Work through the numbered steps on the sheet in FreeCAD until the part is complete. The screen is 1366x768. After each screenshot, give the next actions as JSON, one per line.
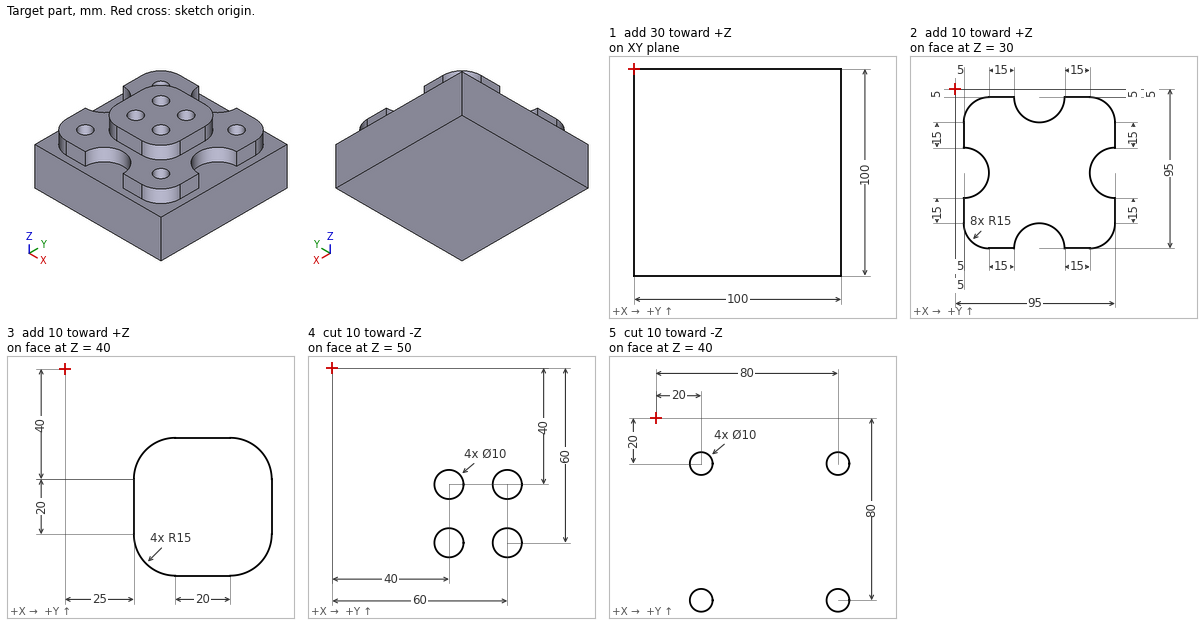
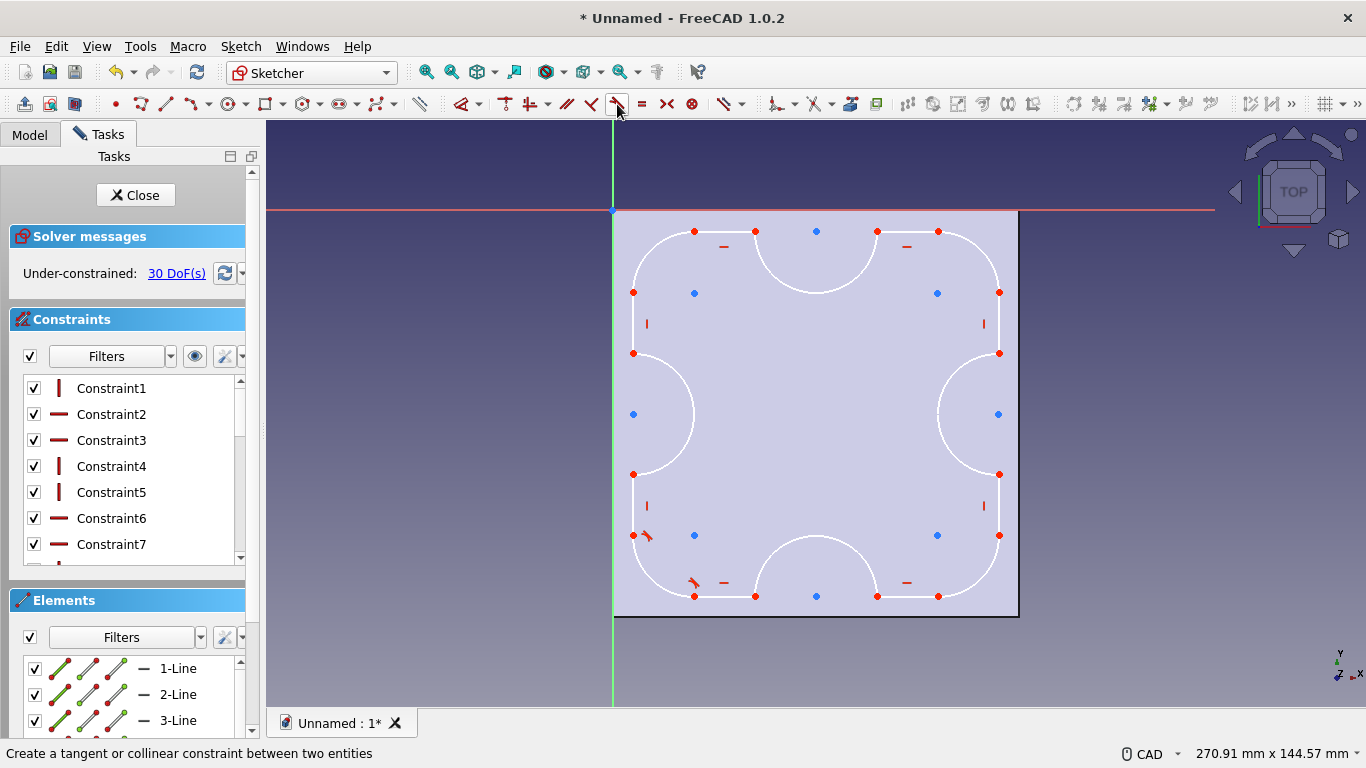
{"action": "left_click", "coordinate": [895, 597]}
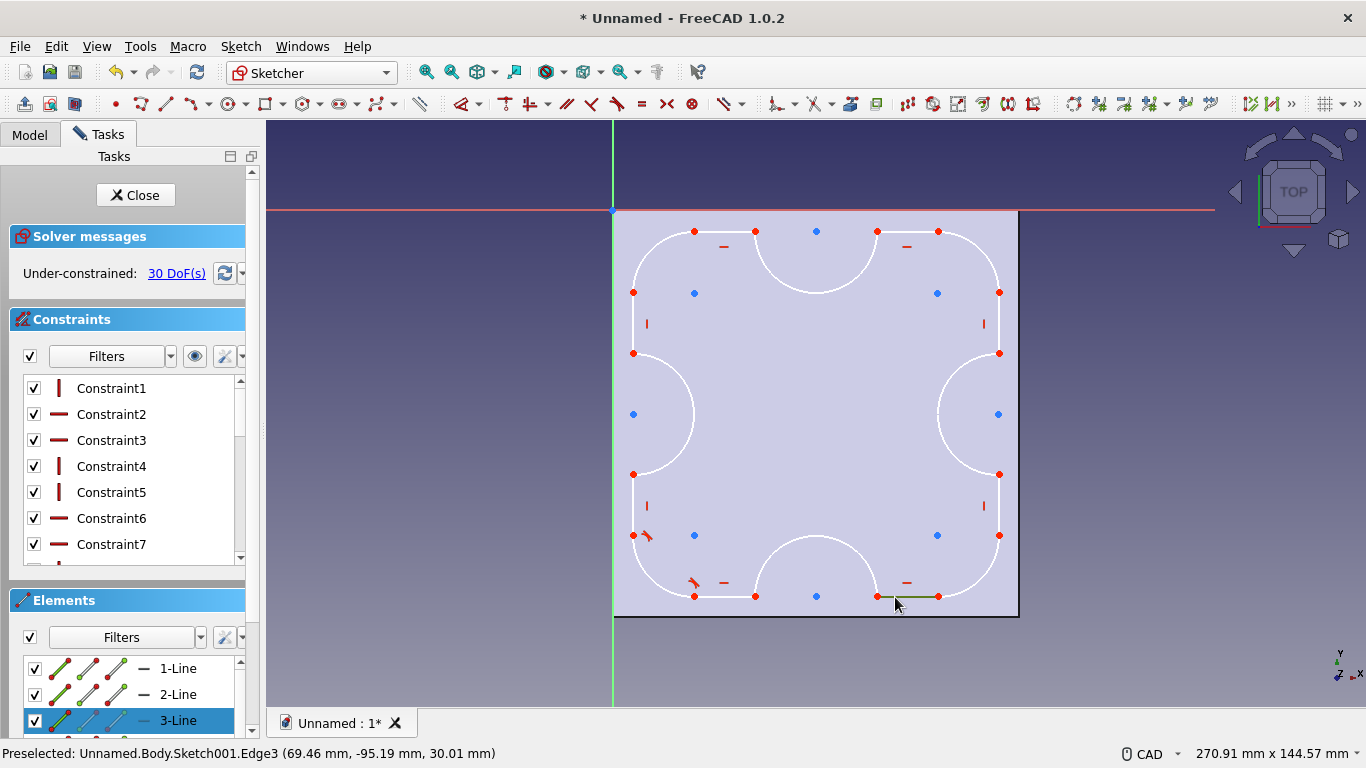
{"action": "left_click", "coordinate": [966, 590]}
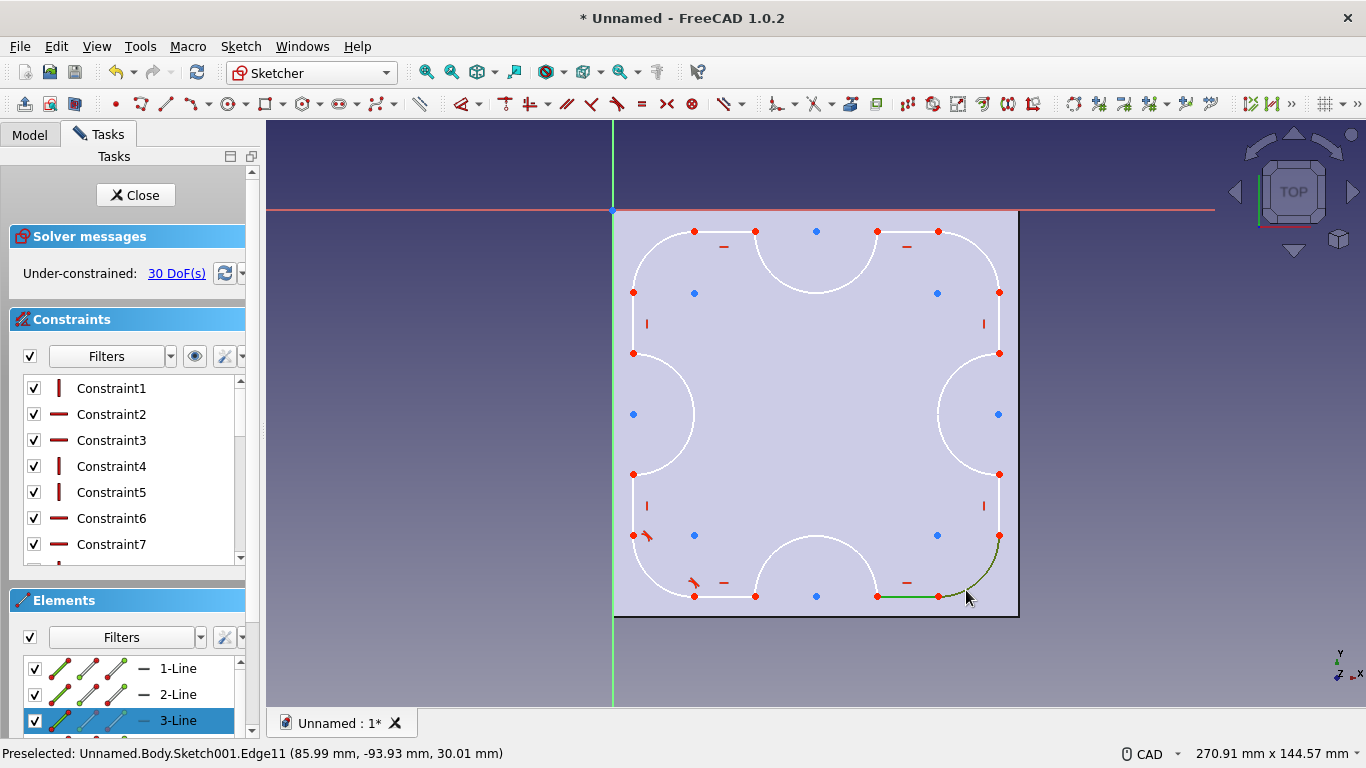
{"action": "left_click", "coordinate": [617, 104]}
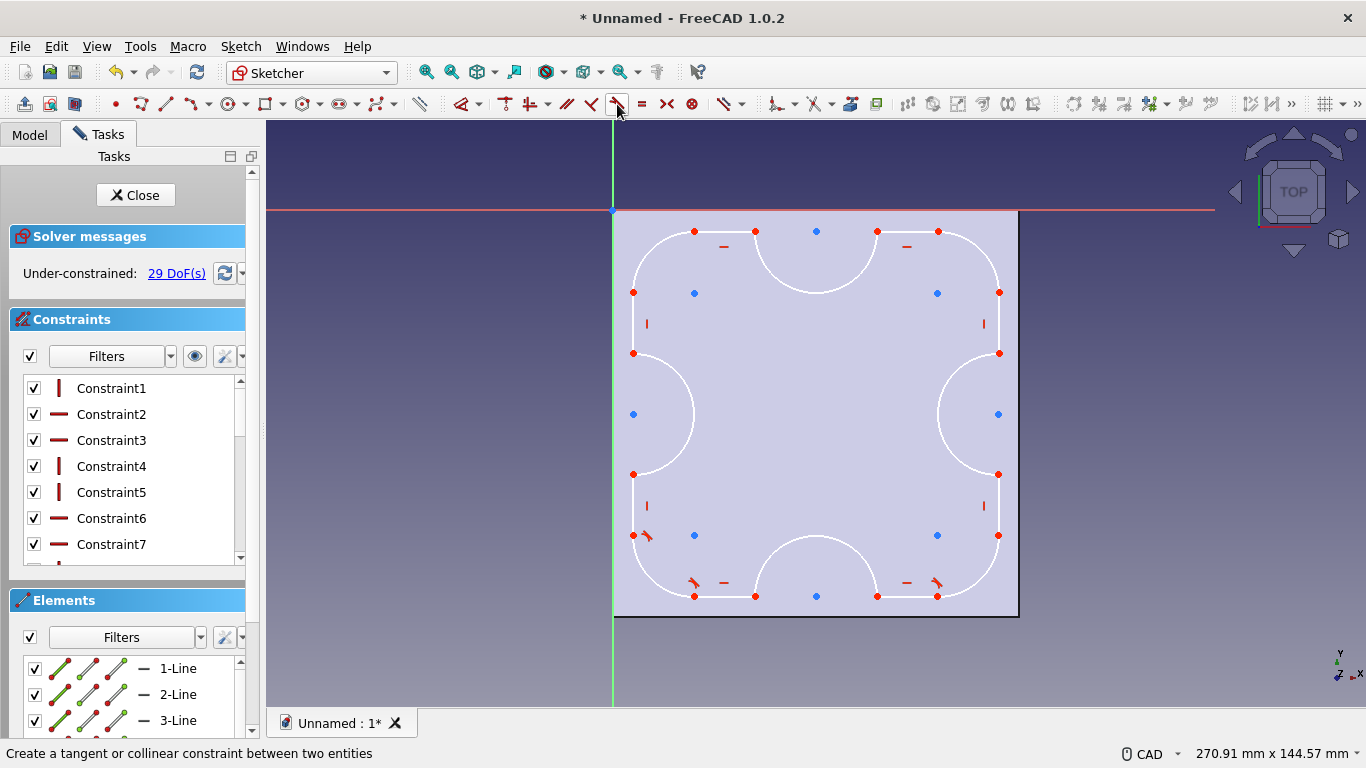
{"action": "left_click", "coordinate": [999, 518]}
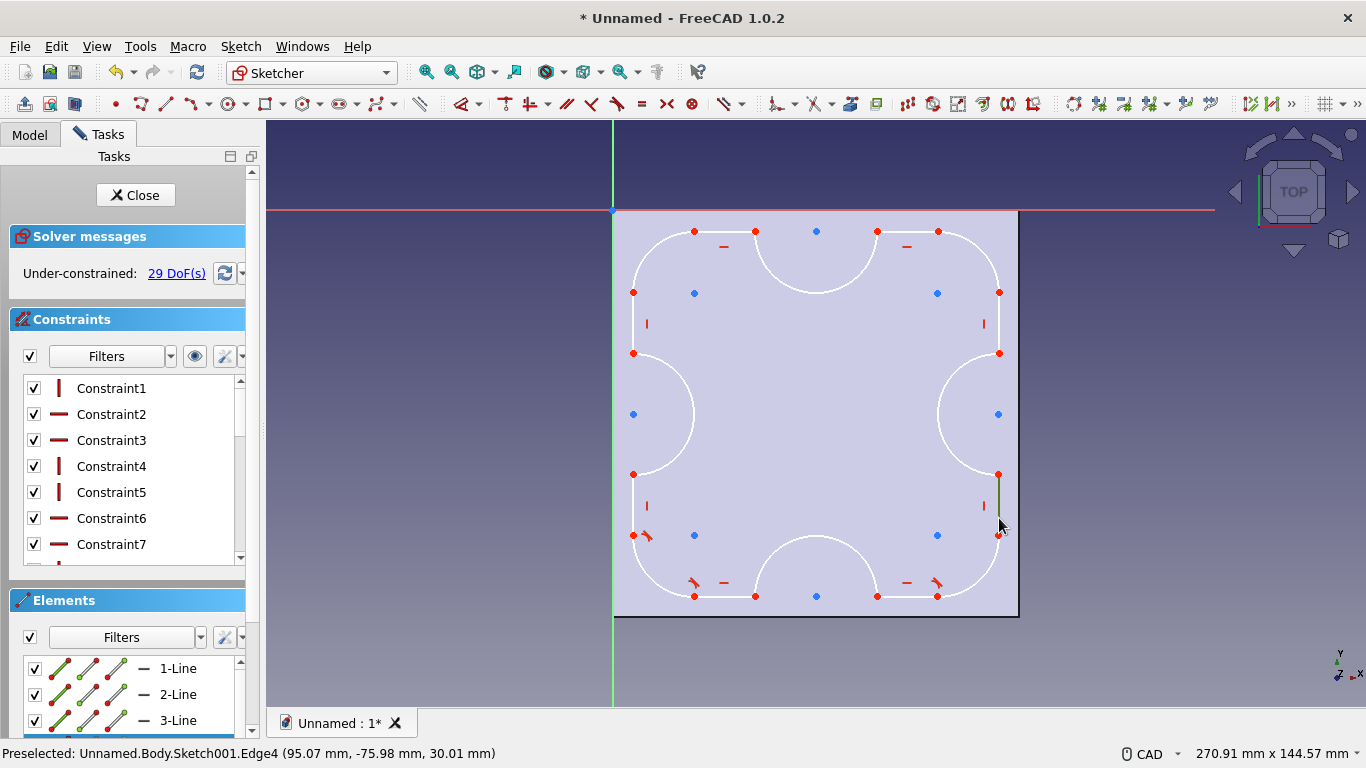
{"action": "left_click", "coordinate": [965, 590]}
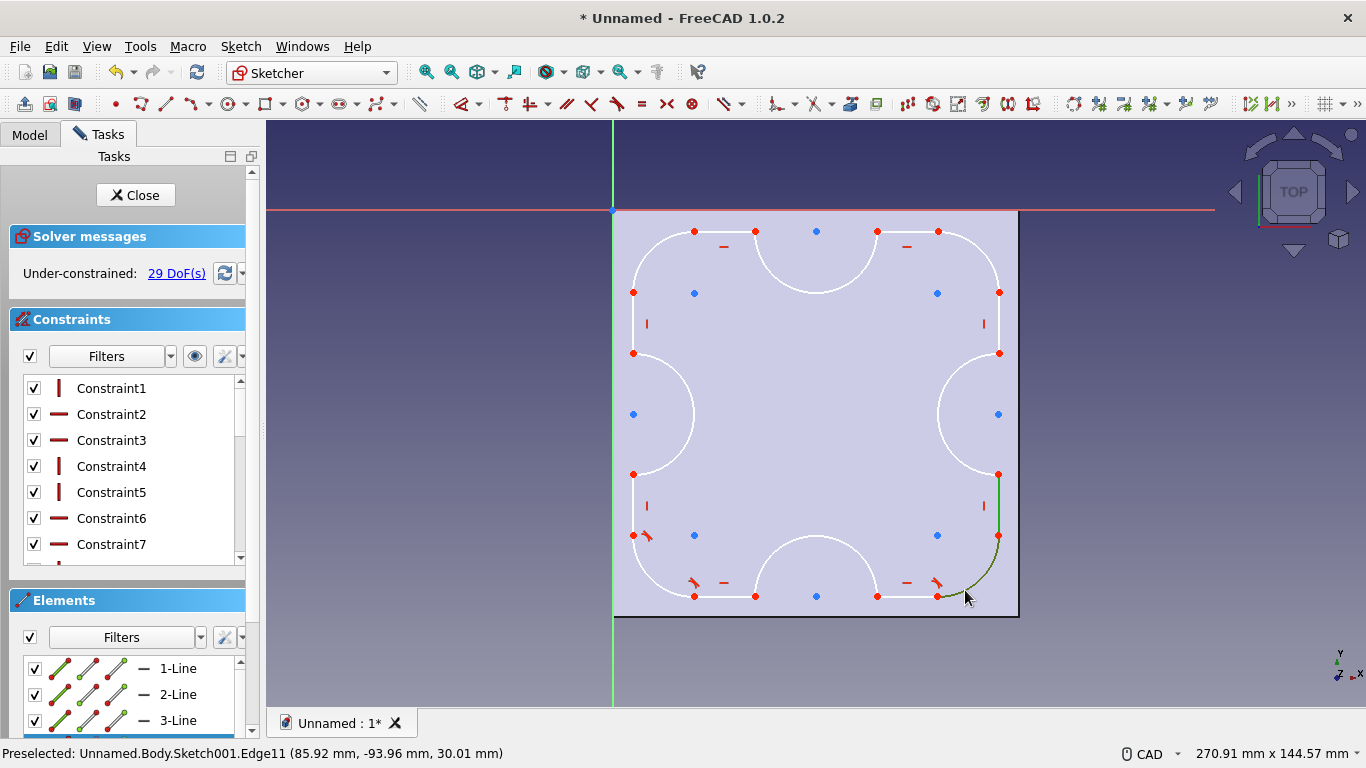
{"action": "left_click", "coordinate": [617, 104]}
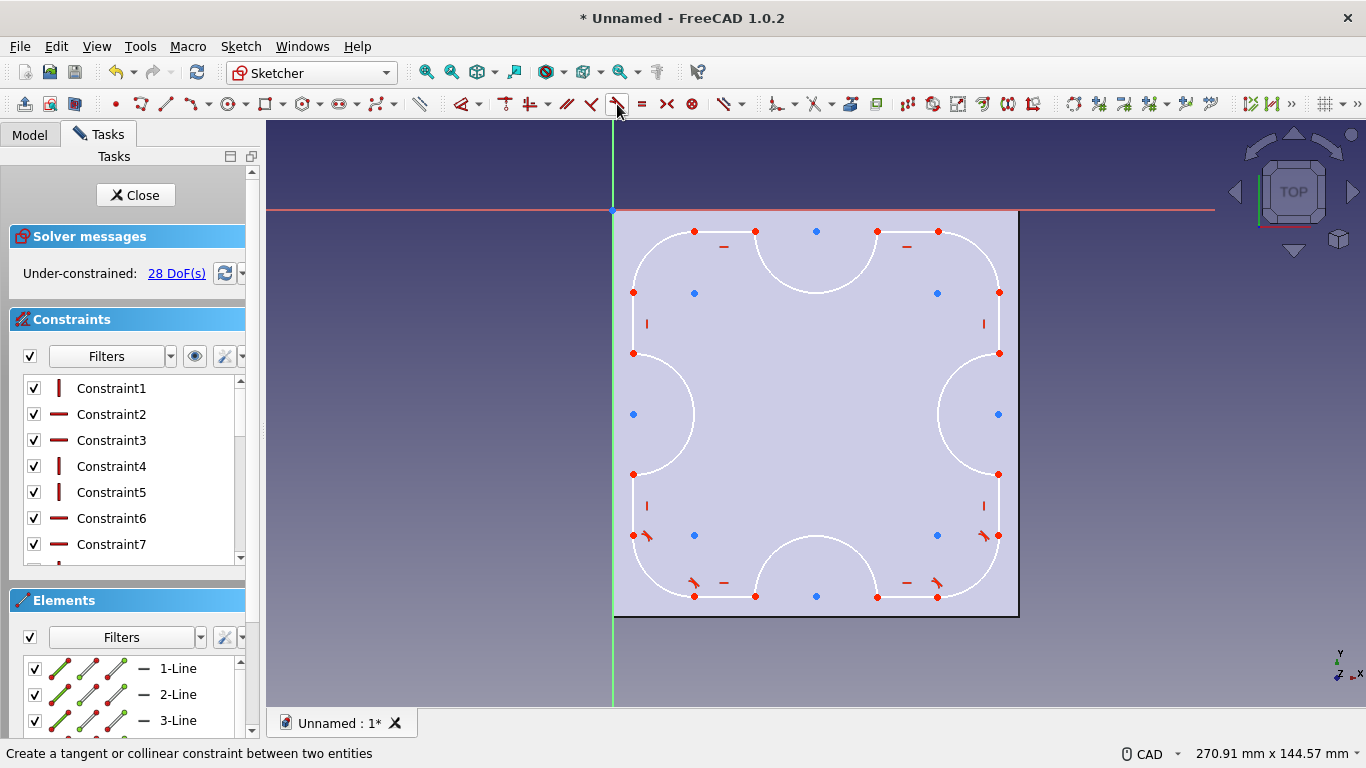
{"action": "left_click", "coordinate": [999, 336]}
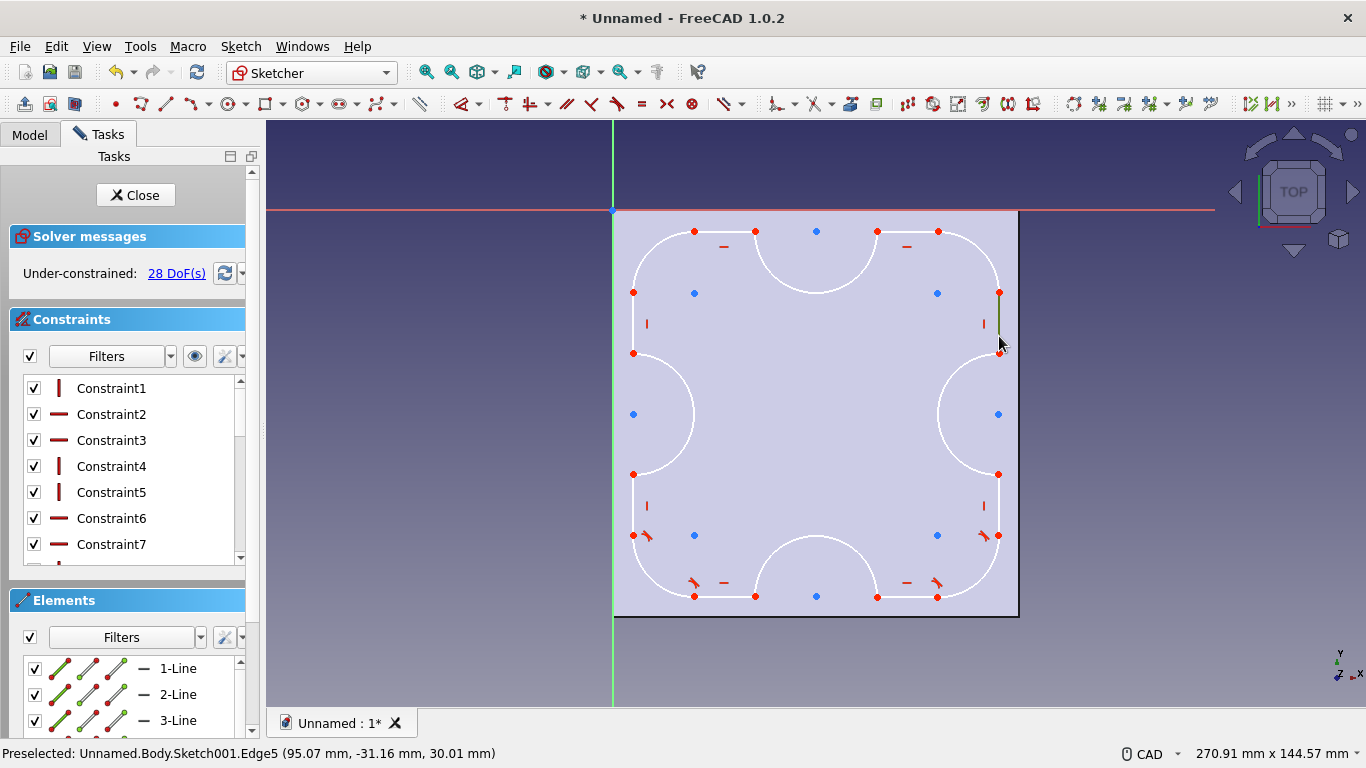
{"action": "left_click", "coordinate": [992, 265]}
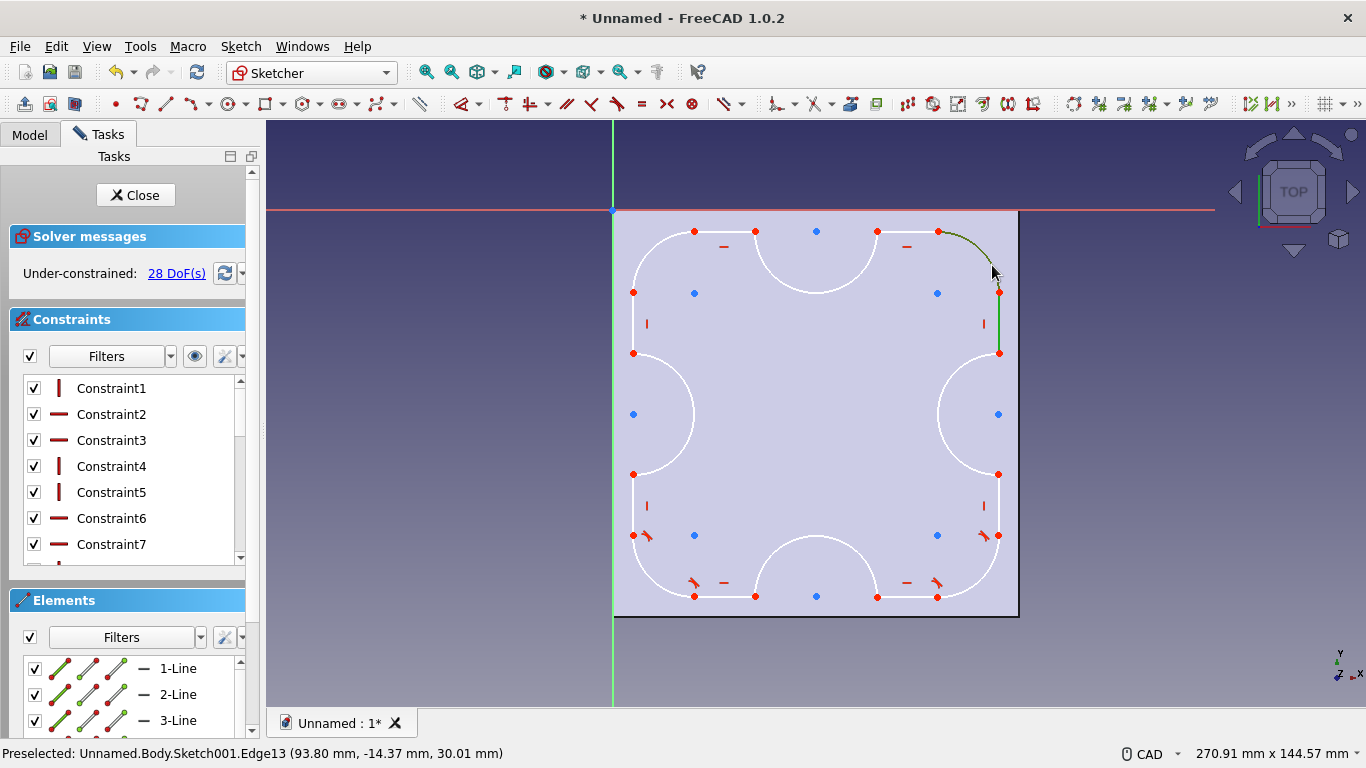
{"action": "left_click", "coordinate": [617, 104]}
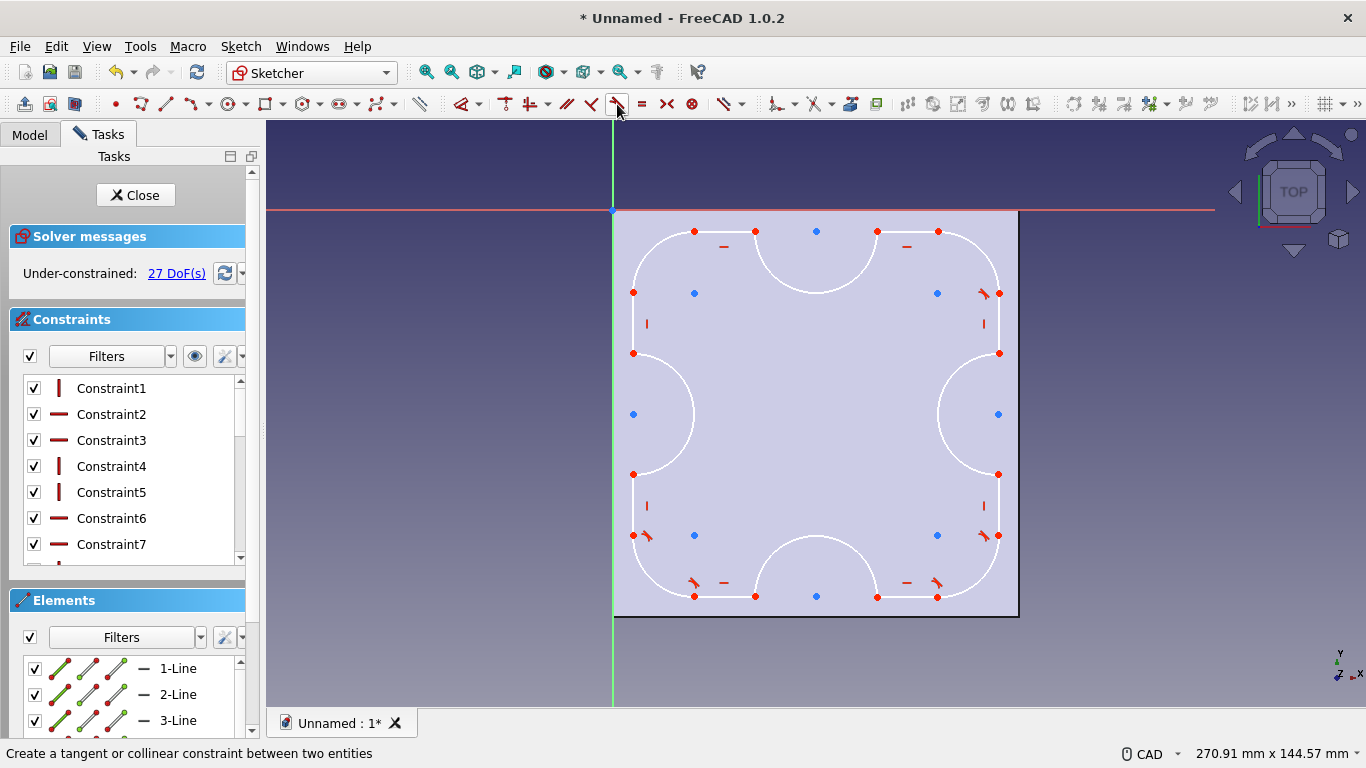
{"action": "left_click", "coordinate": [920, 232]}